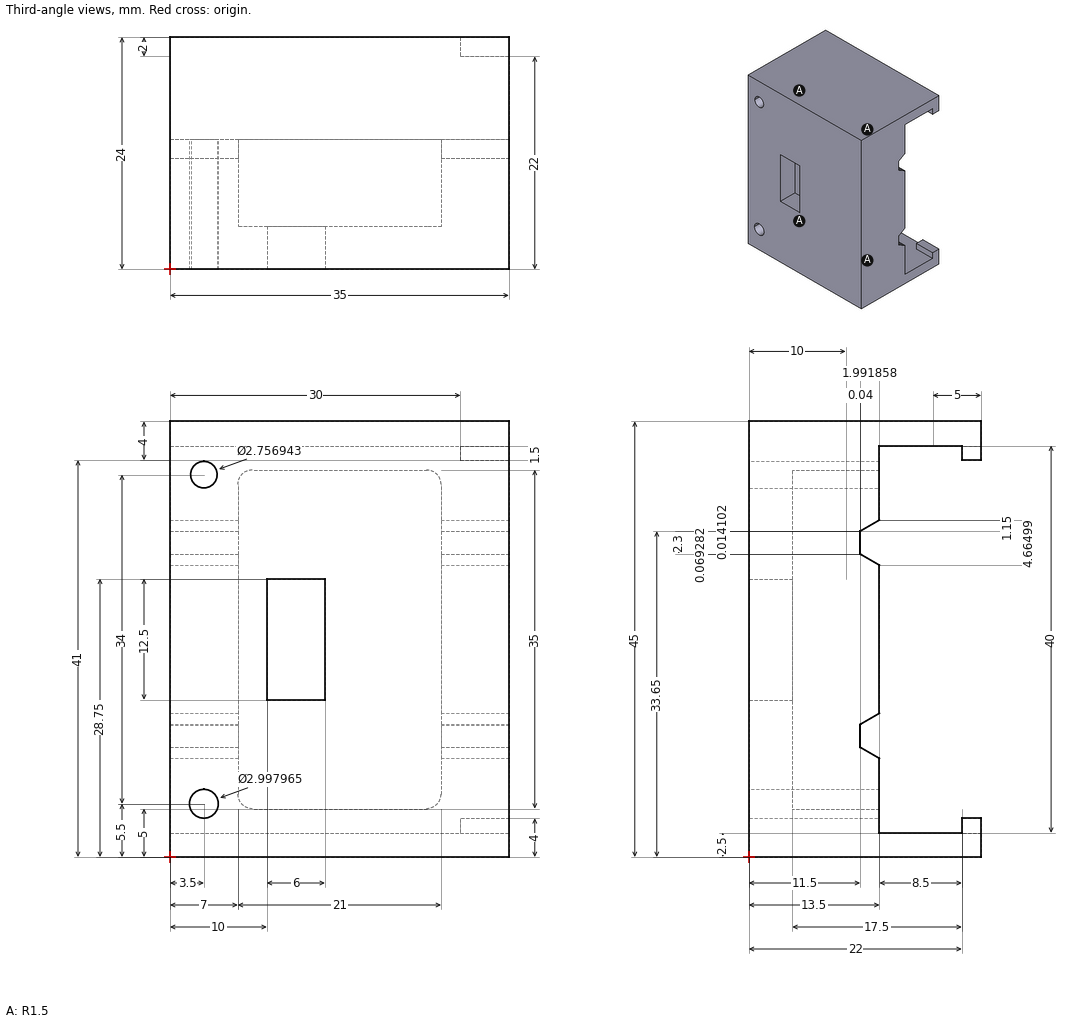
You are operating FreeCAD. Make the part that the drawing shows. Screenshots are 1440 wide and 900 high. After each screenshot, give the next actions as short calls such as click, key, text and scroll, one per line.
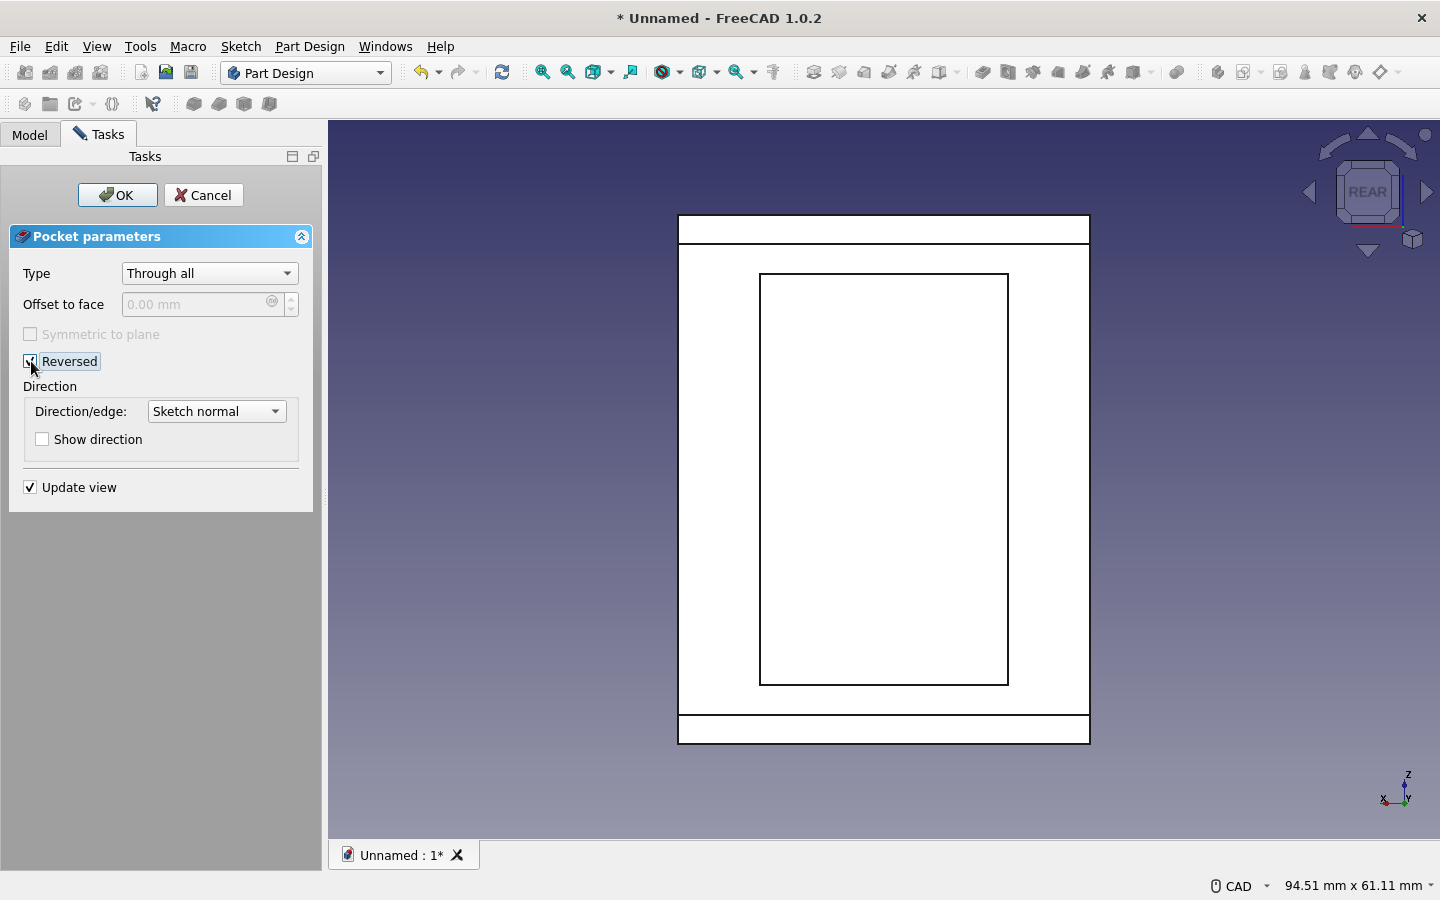
click(118, 195)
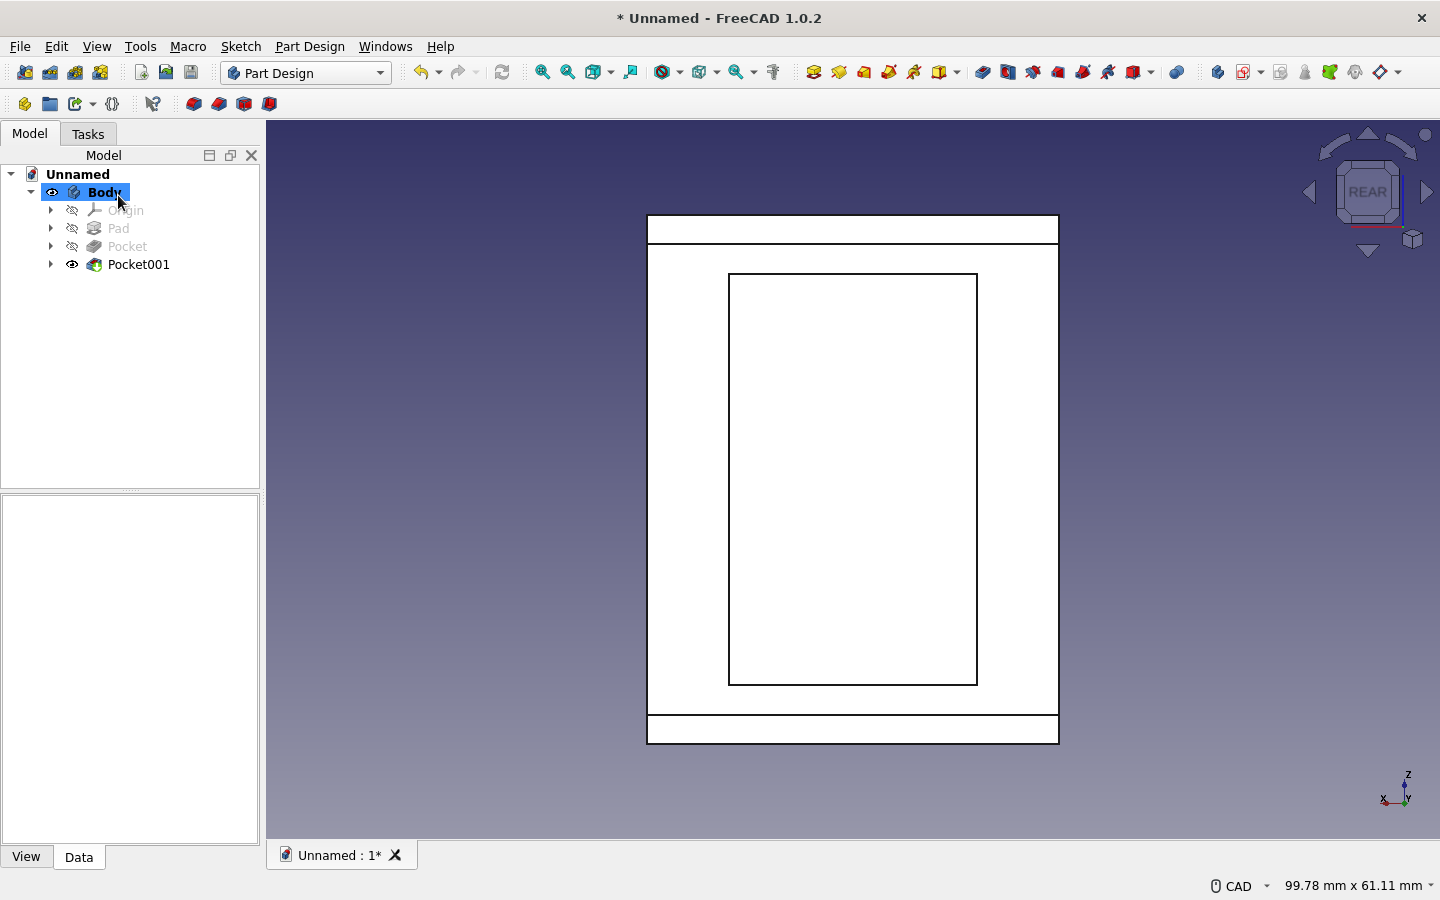
key(0)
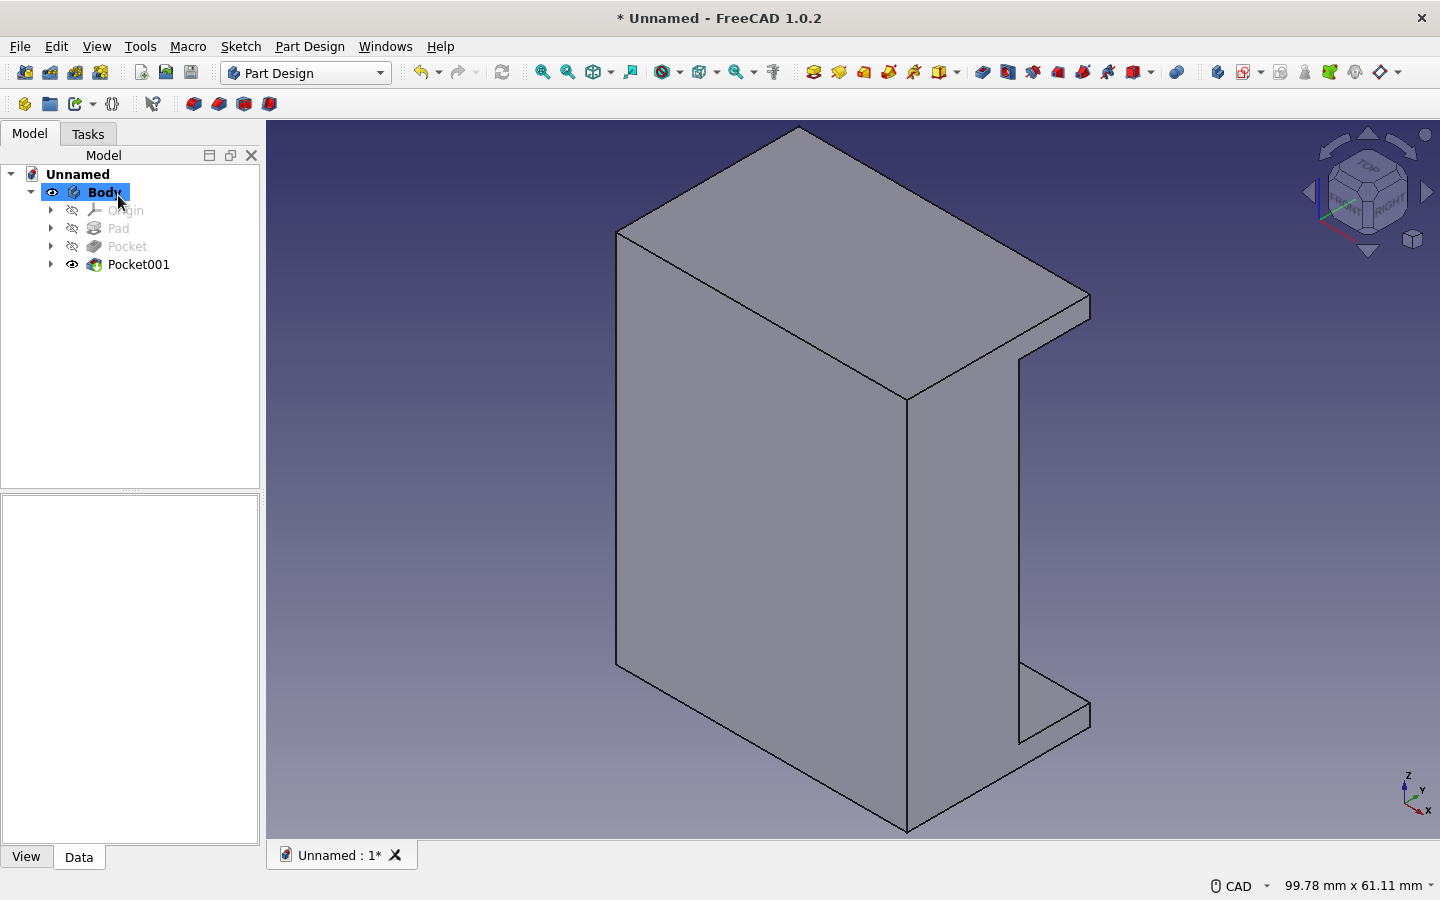
key(2)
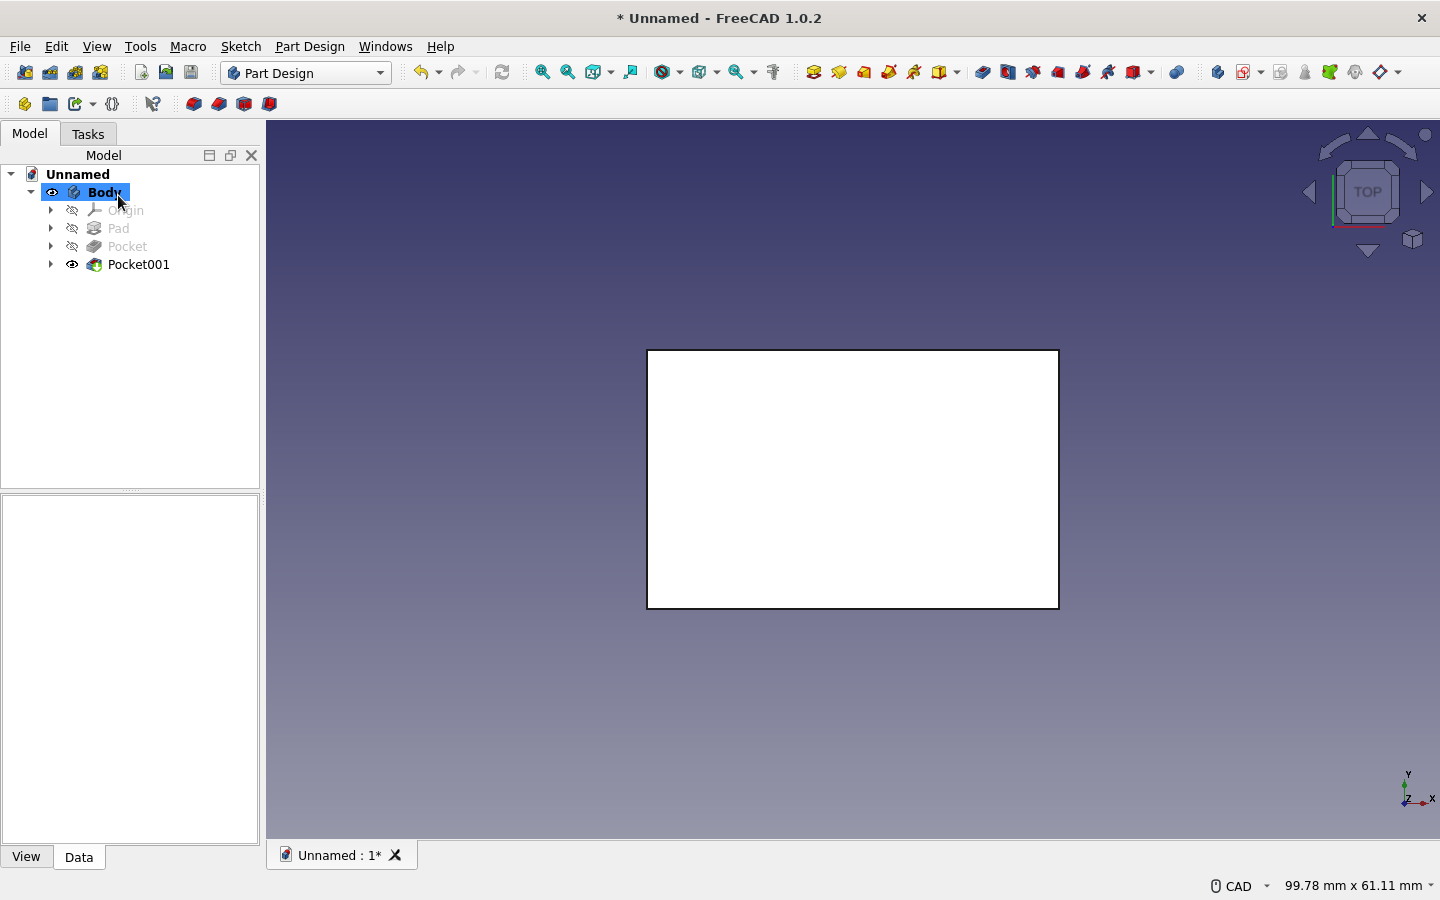
click(543, 72)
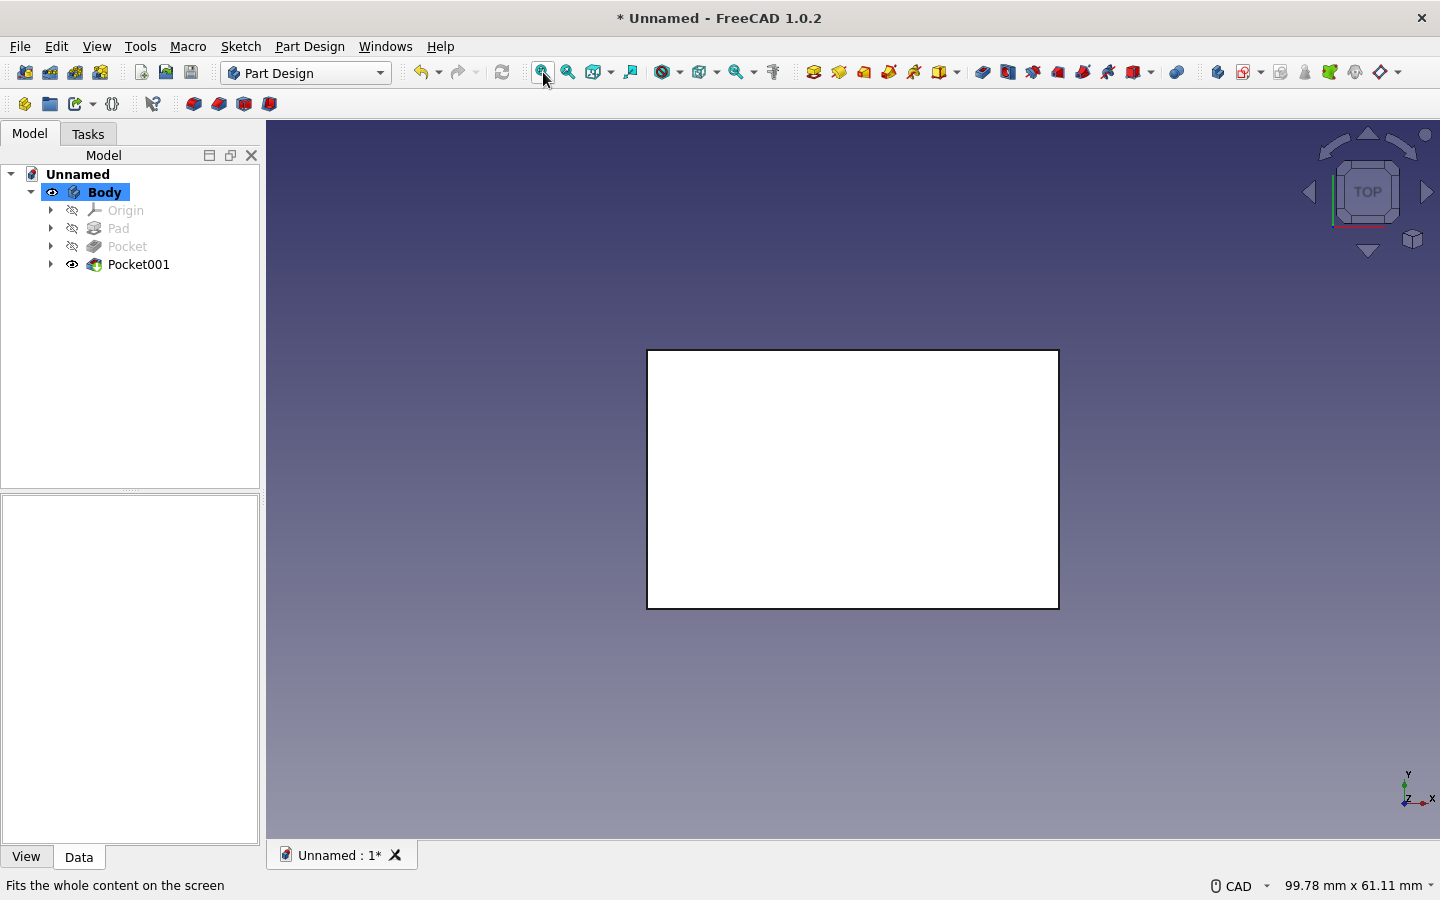
key(1)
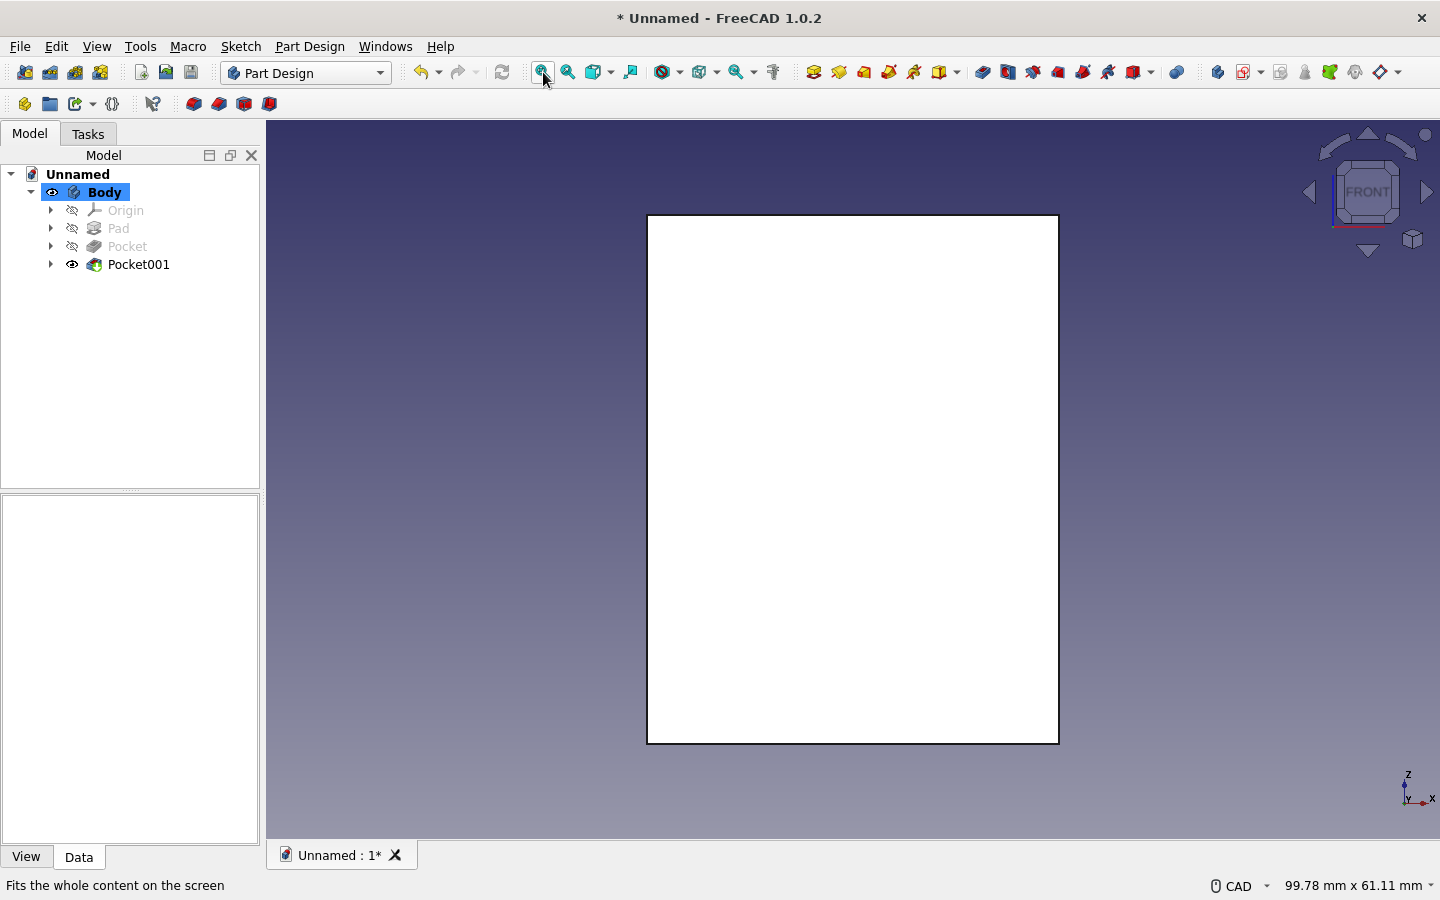
key(3)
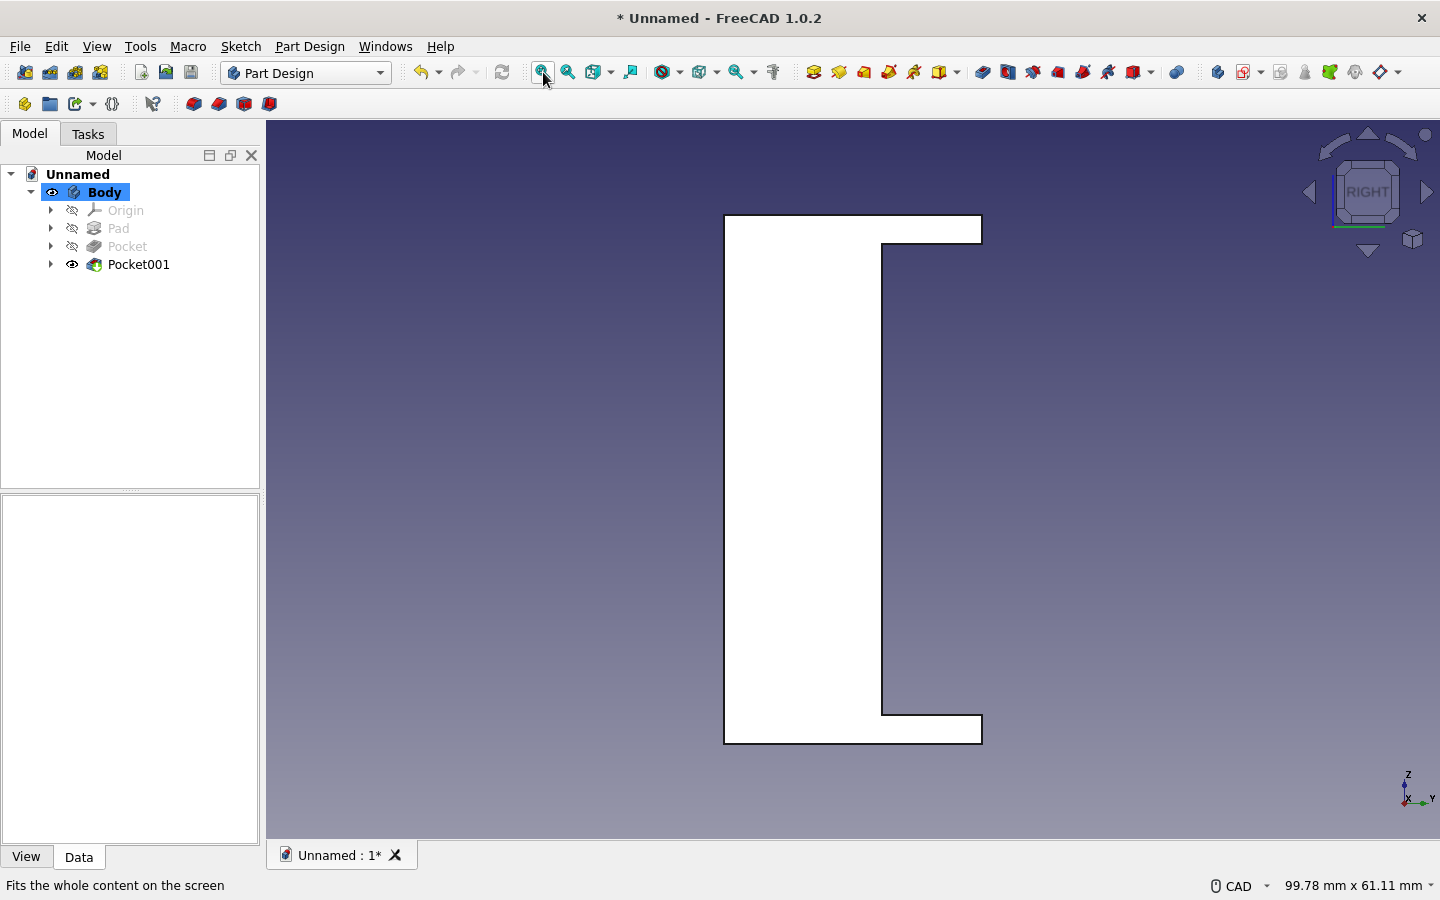
key(5)